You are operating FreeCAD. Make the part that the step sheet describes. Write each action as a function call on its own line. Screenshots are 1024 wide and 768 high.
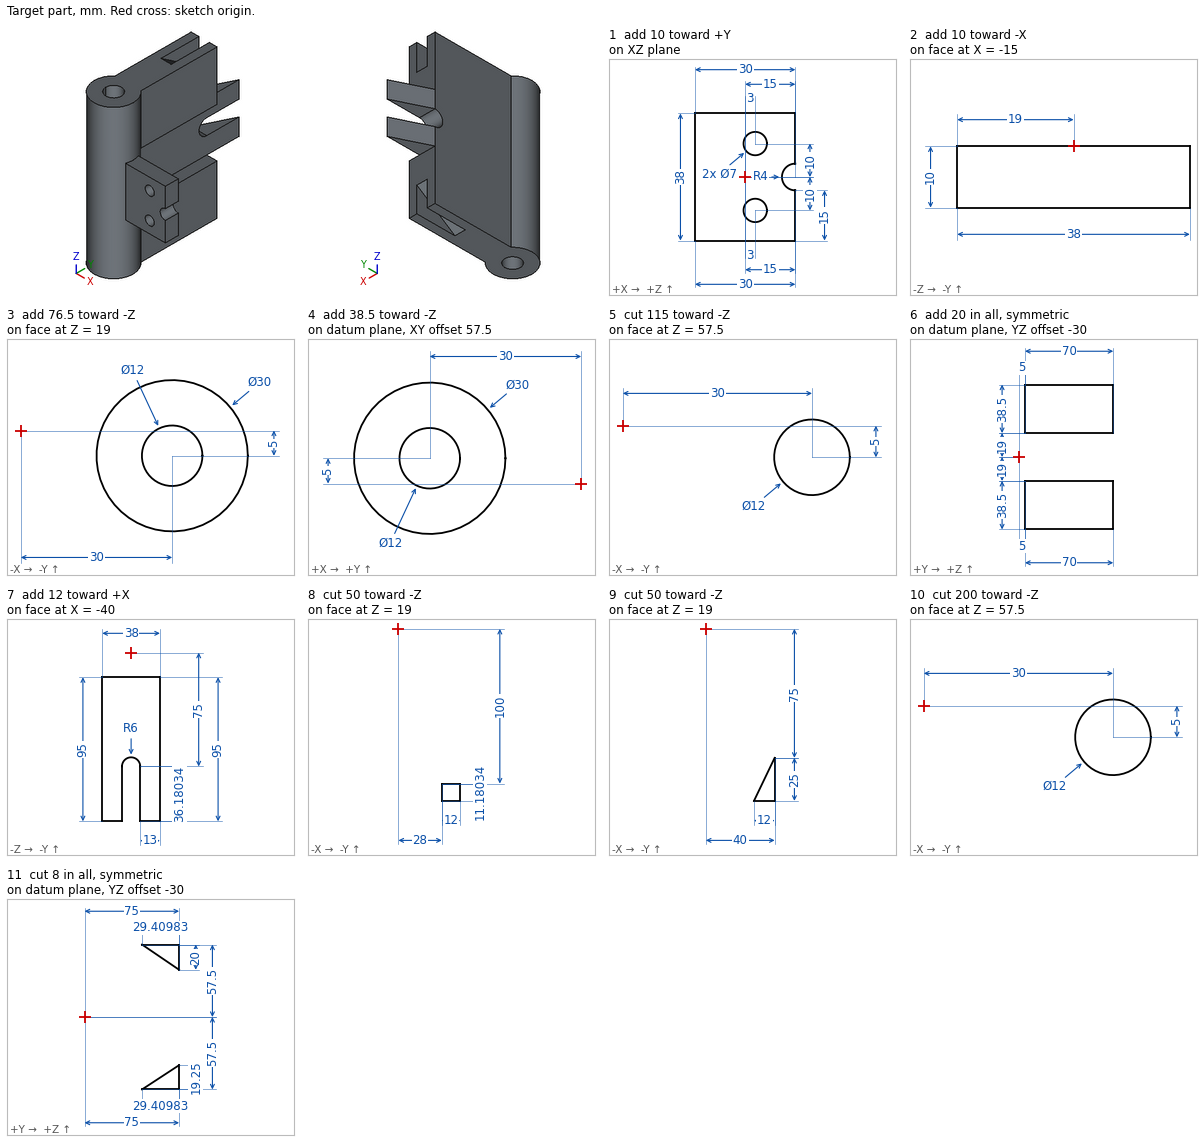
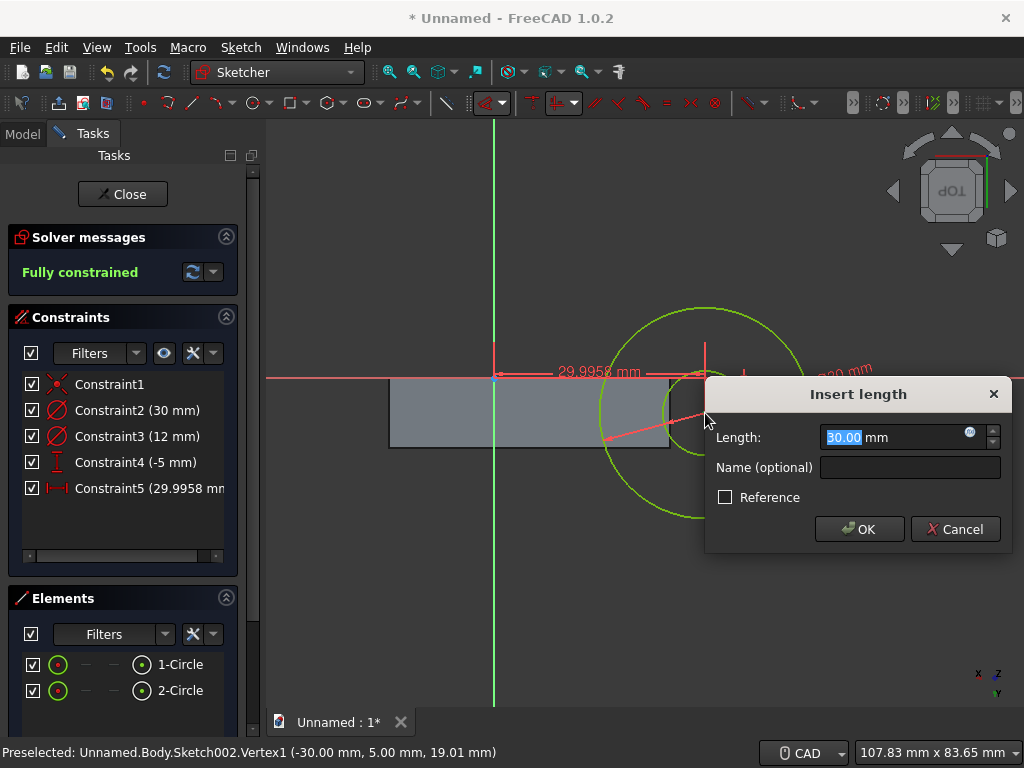
text(30)
key(Return)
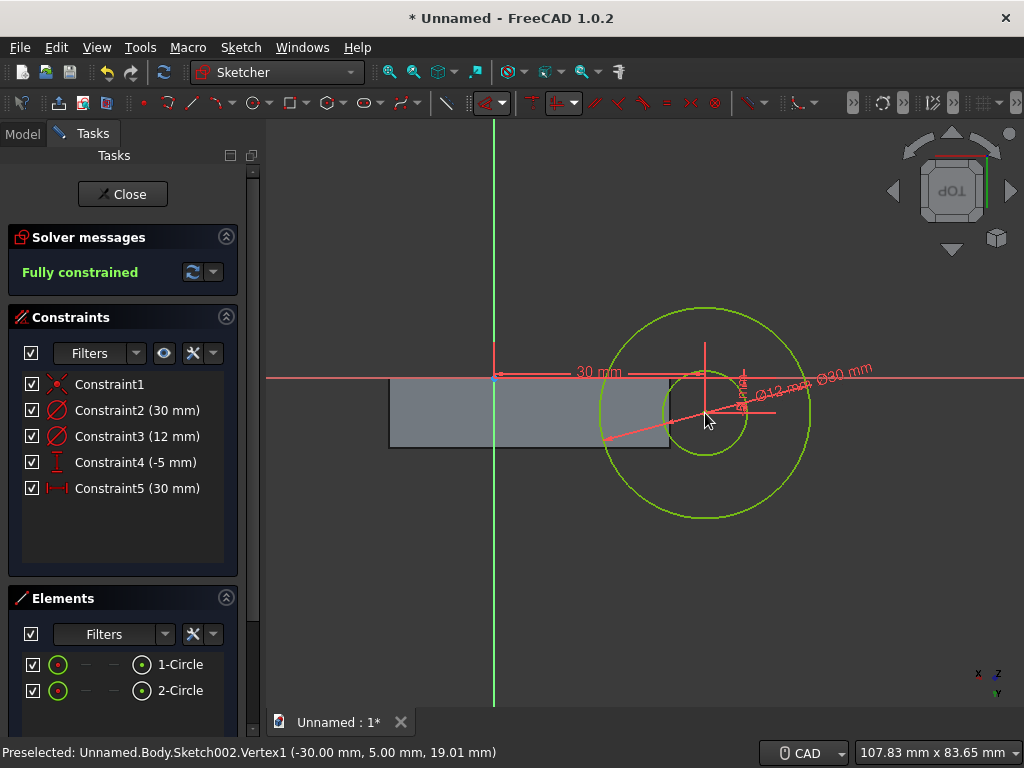
click(123, 194)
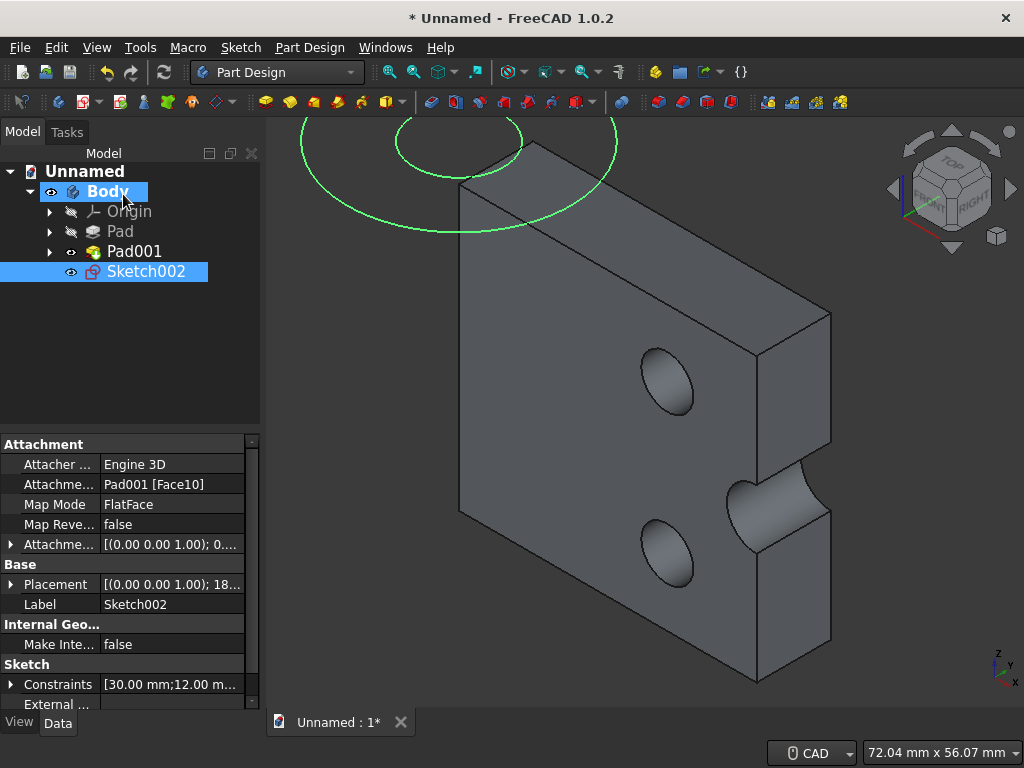
click(266, 102)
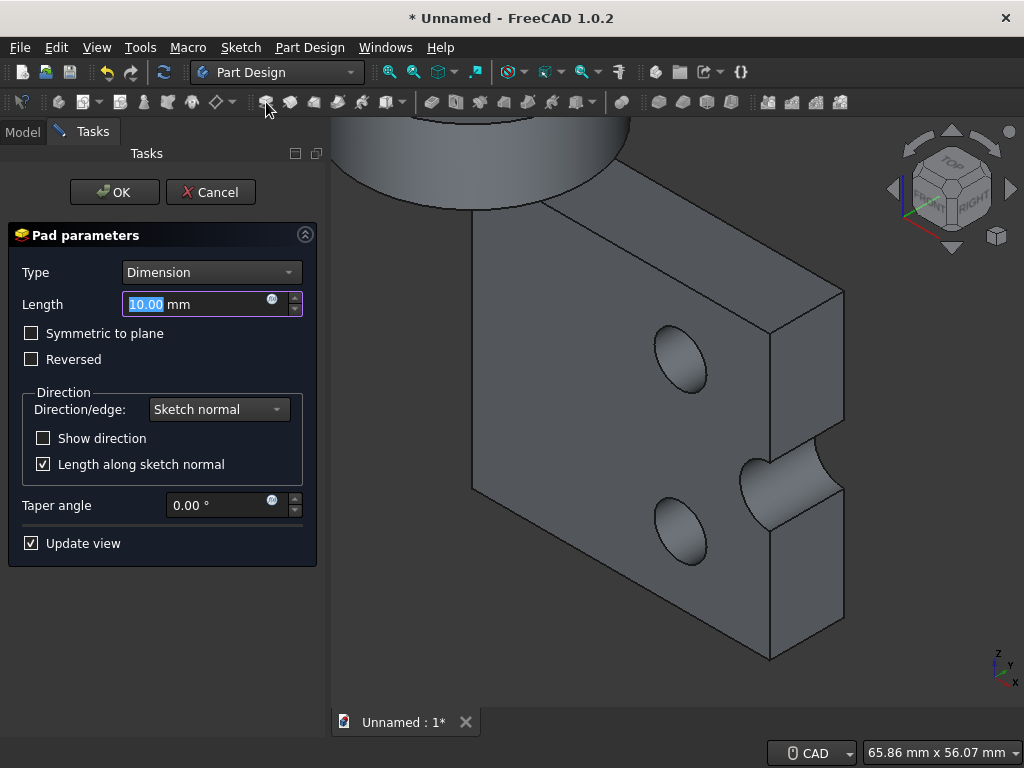
text(76.5)
key(Tab)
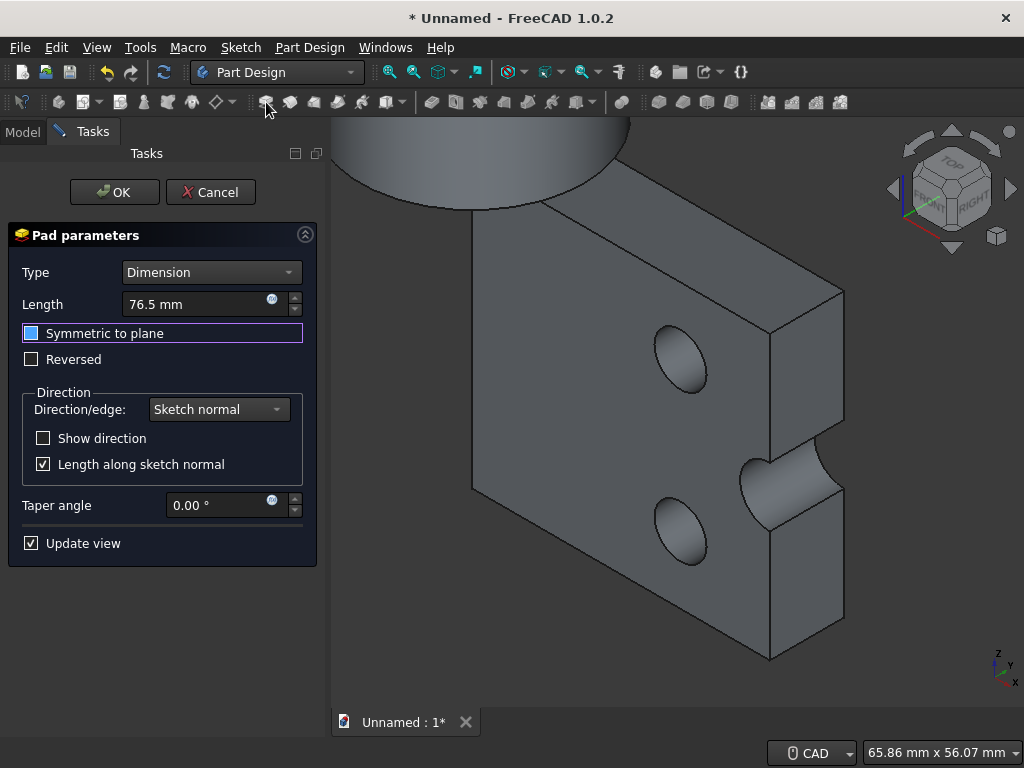
click(30, 359)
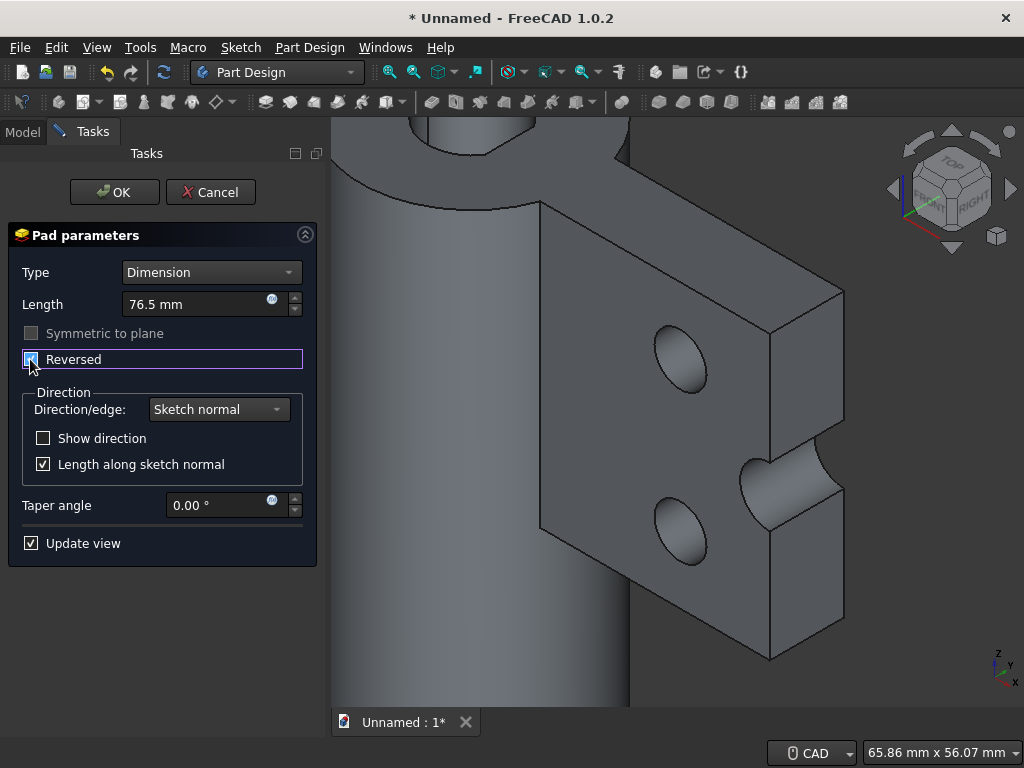
click(115, 192)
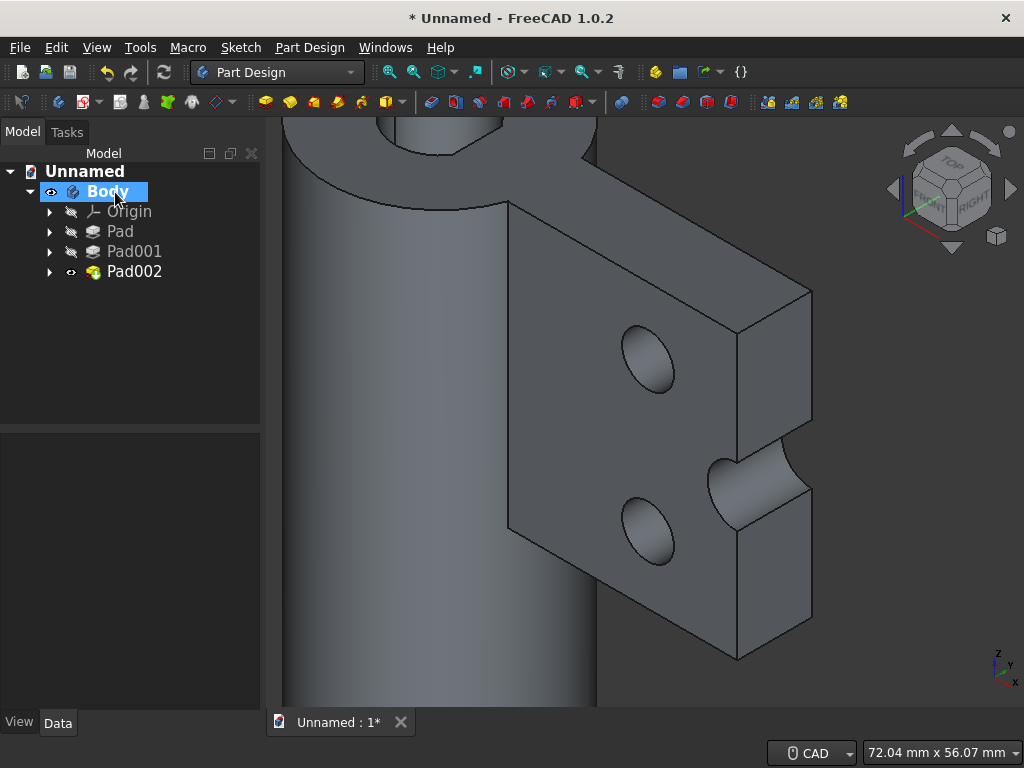
key(v)
key(f)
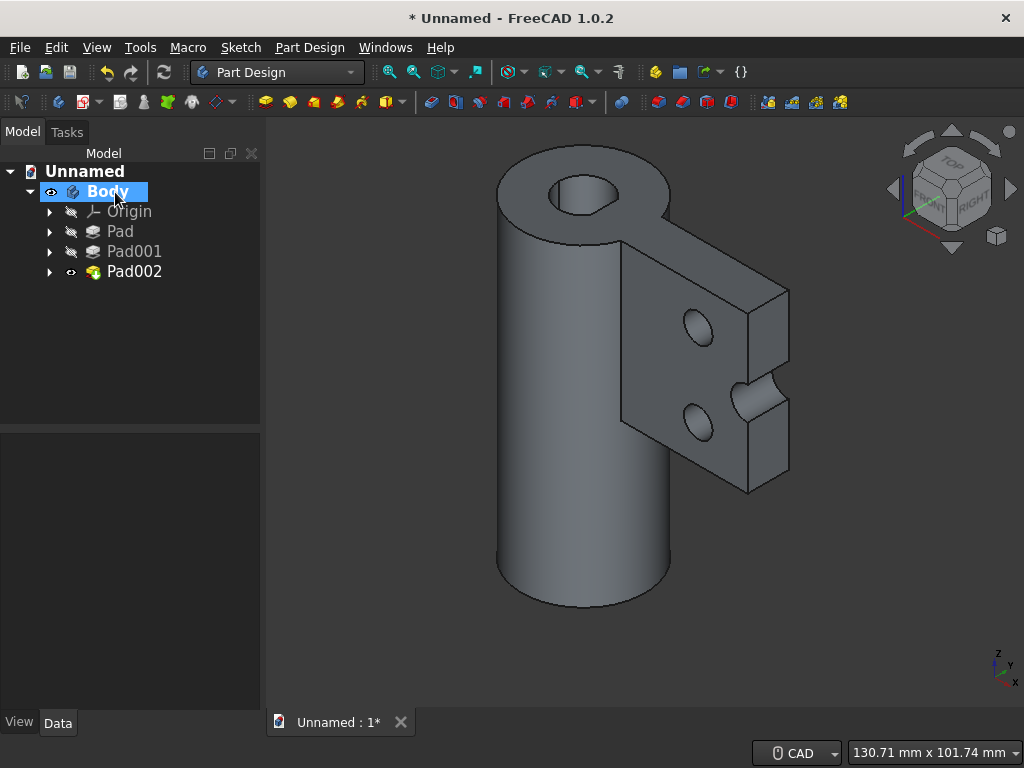
click(50, 212)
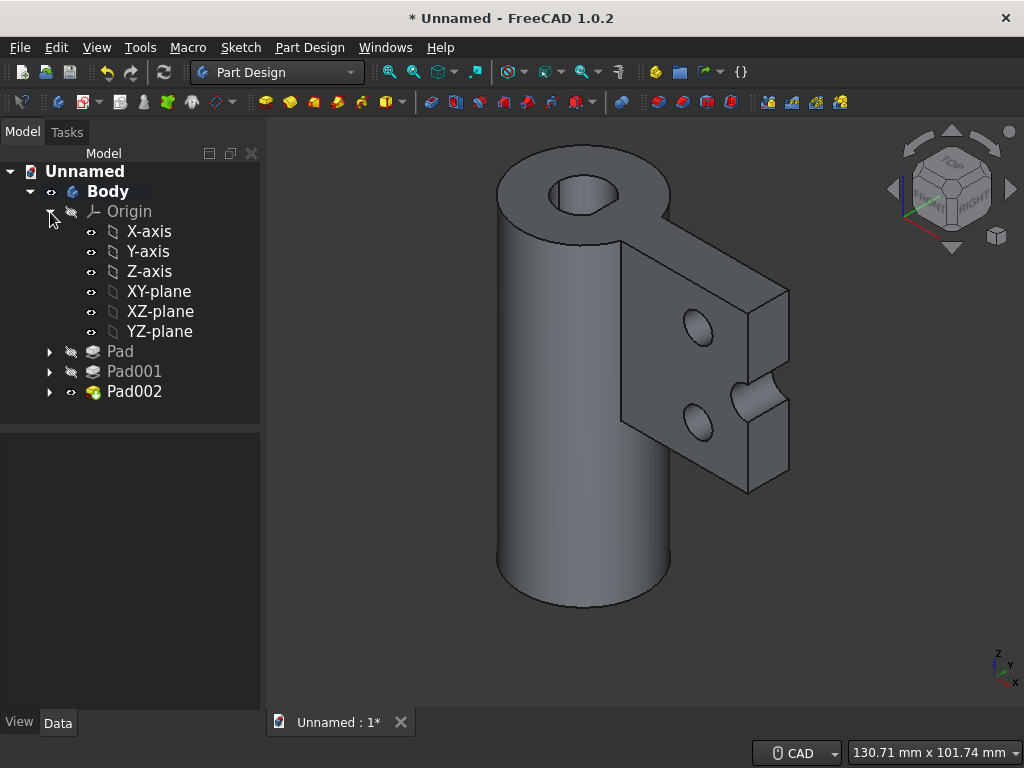
click(136, 292)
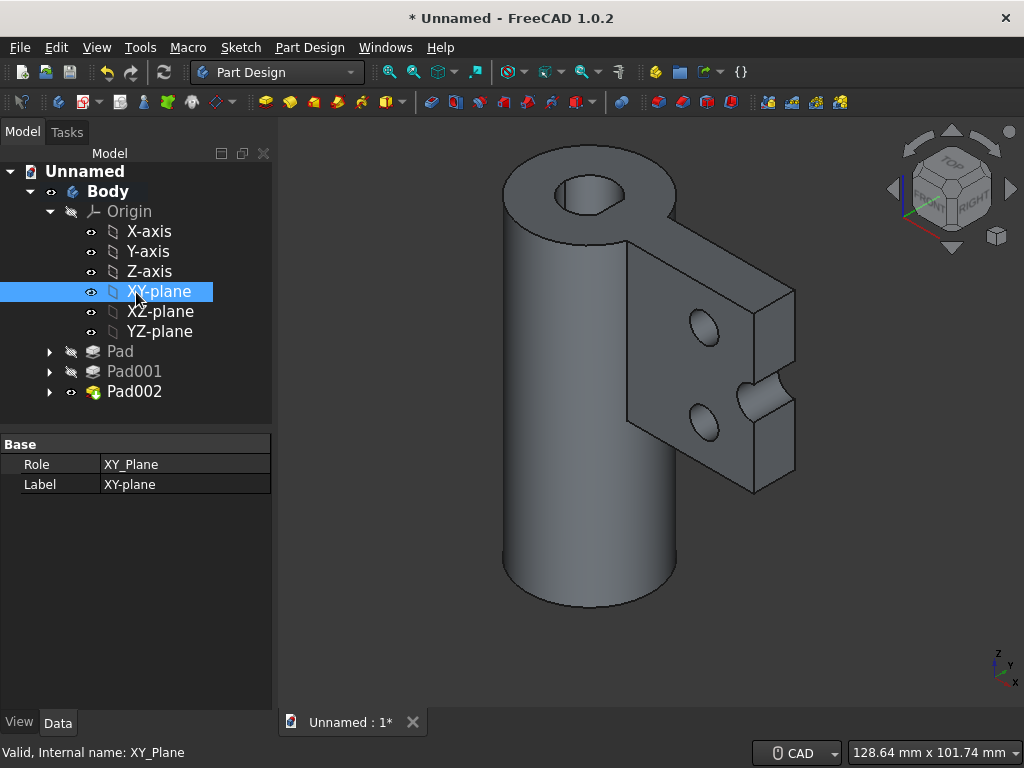
click(216, 102)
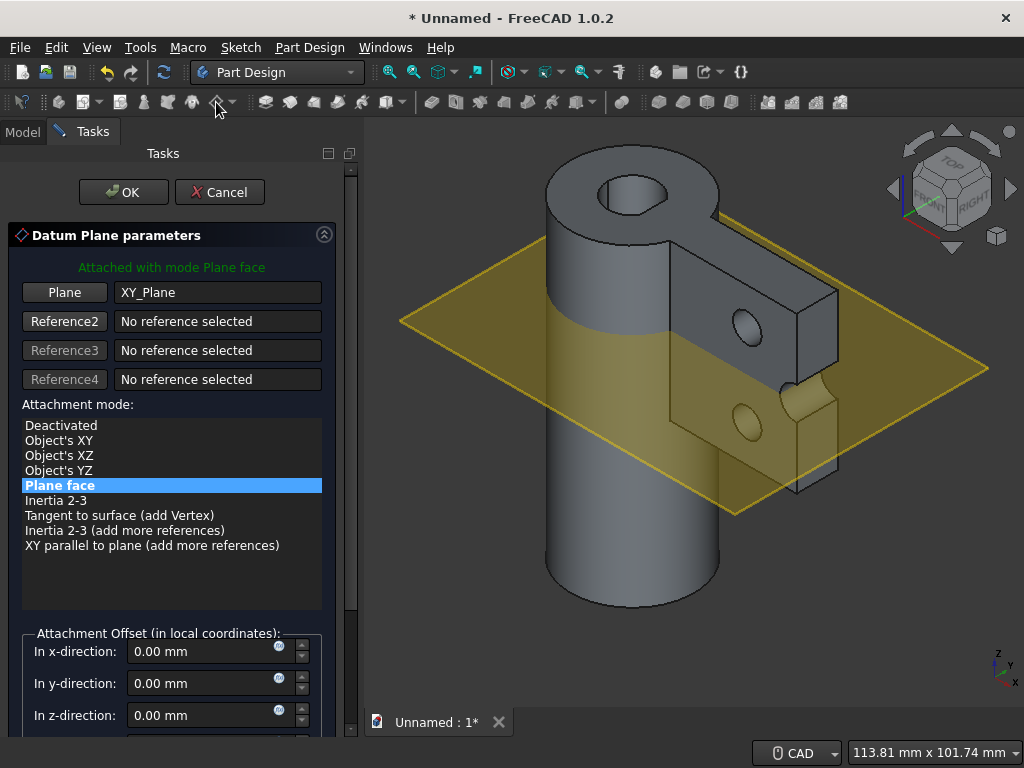
triple_click(210, 715)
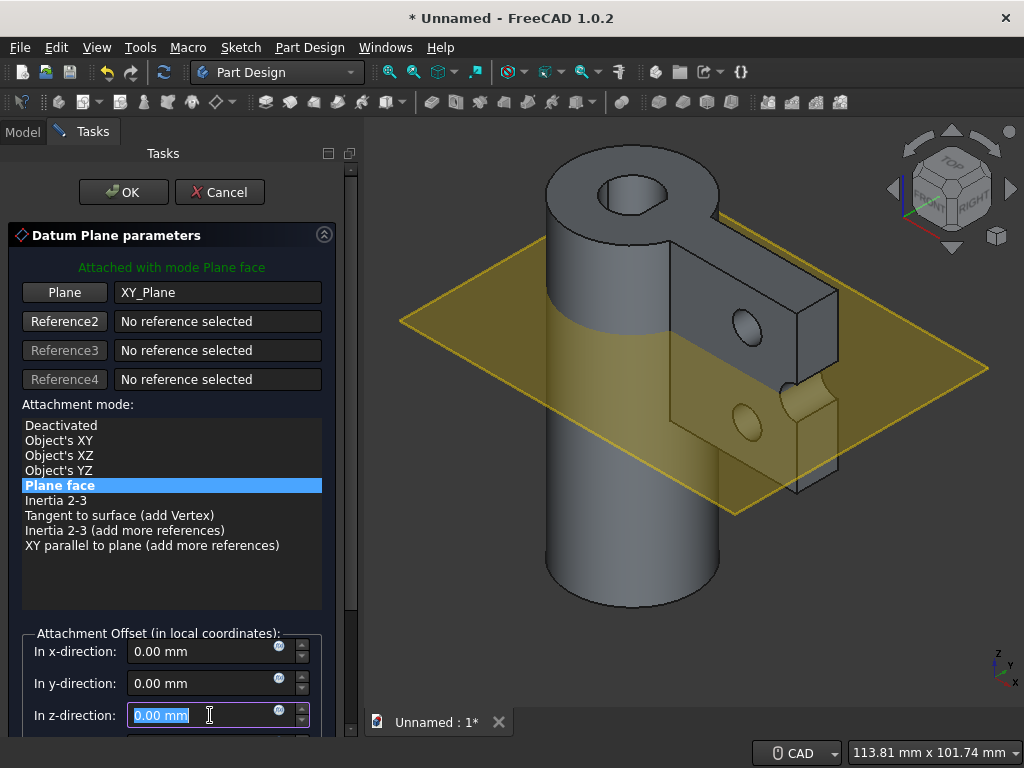
text(57.5)
key(Tab)